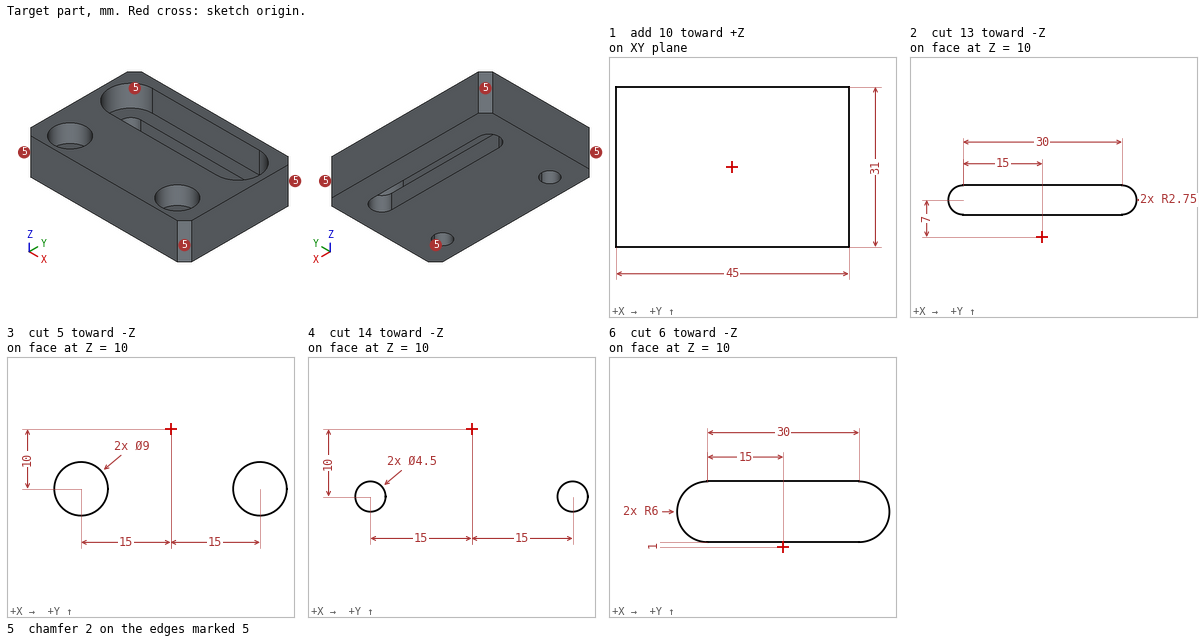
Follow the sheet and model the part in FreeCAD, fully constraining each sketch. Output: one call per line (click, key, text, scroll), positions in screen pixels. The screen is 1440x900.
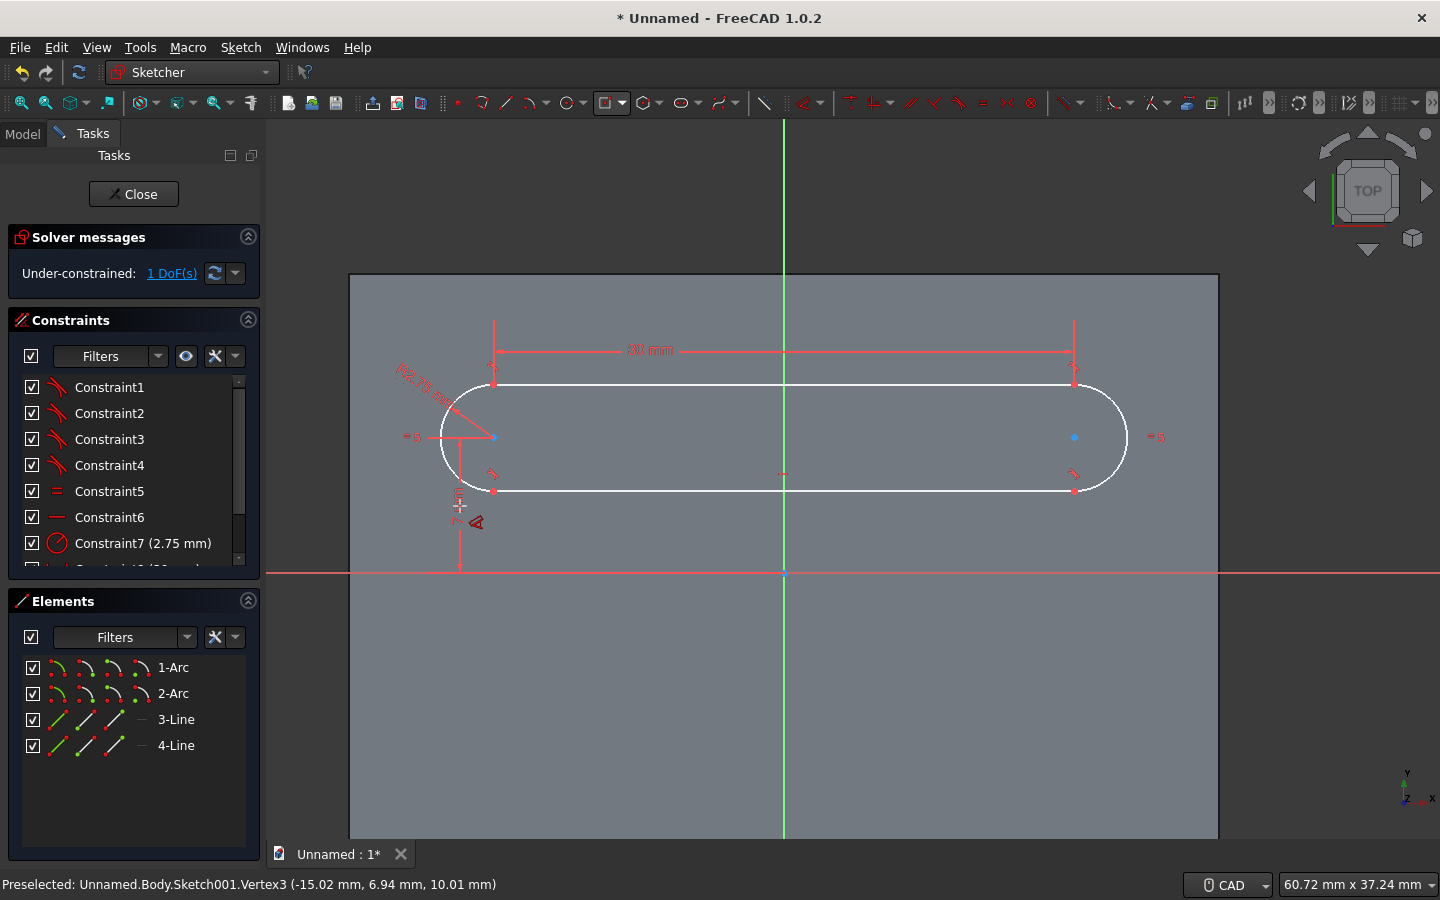
click(494, 385)
click(639, 607)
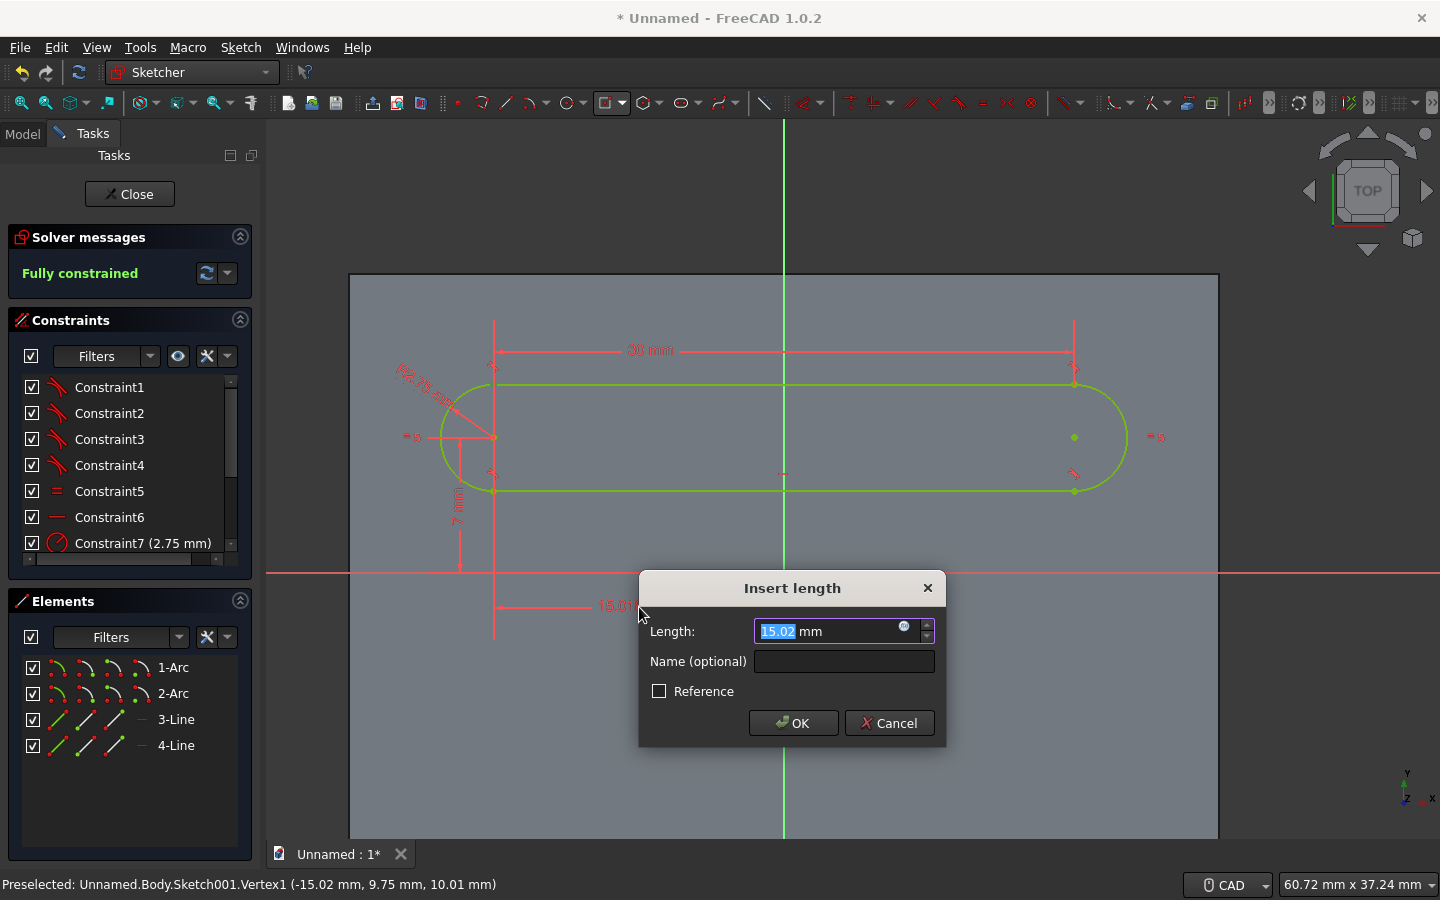
text(15)
key(Return)
key(Escape)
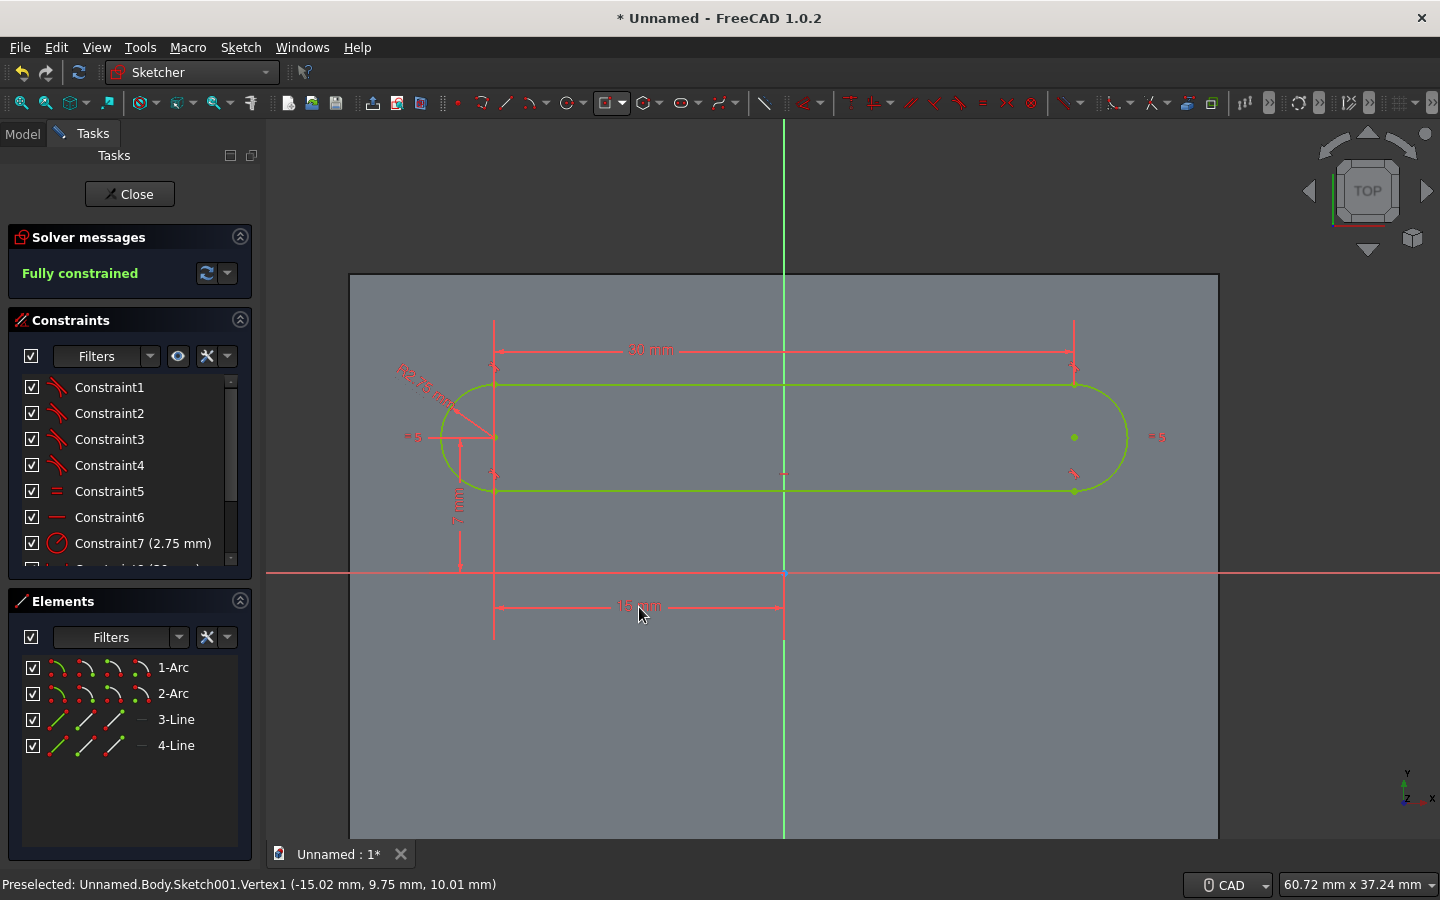
click(130, 194)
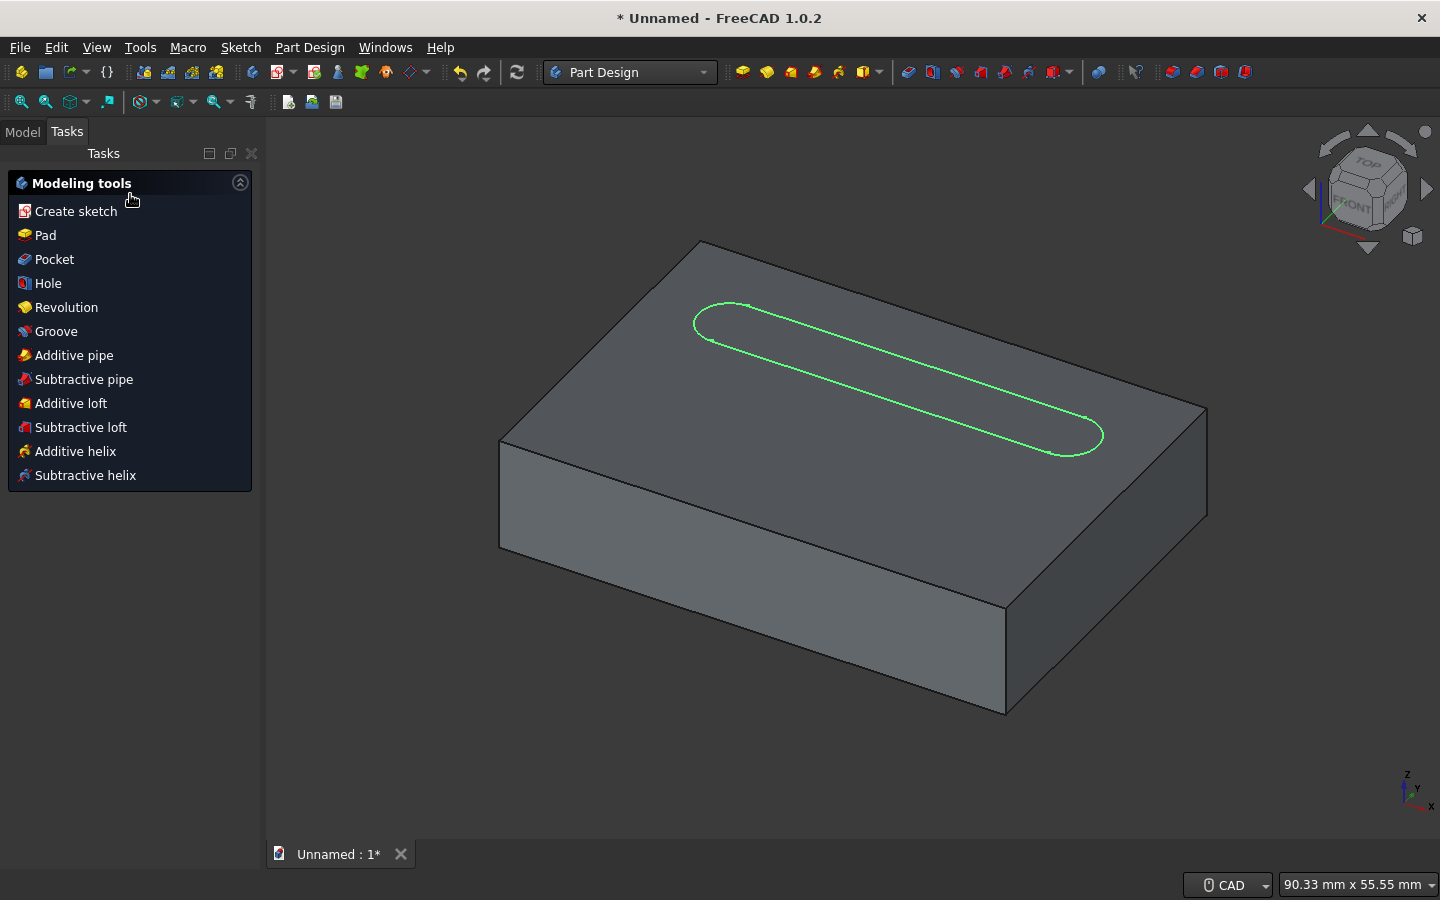
click(910, 72)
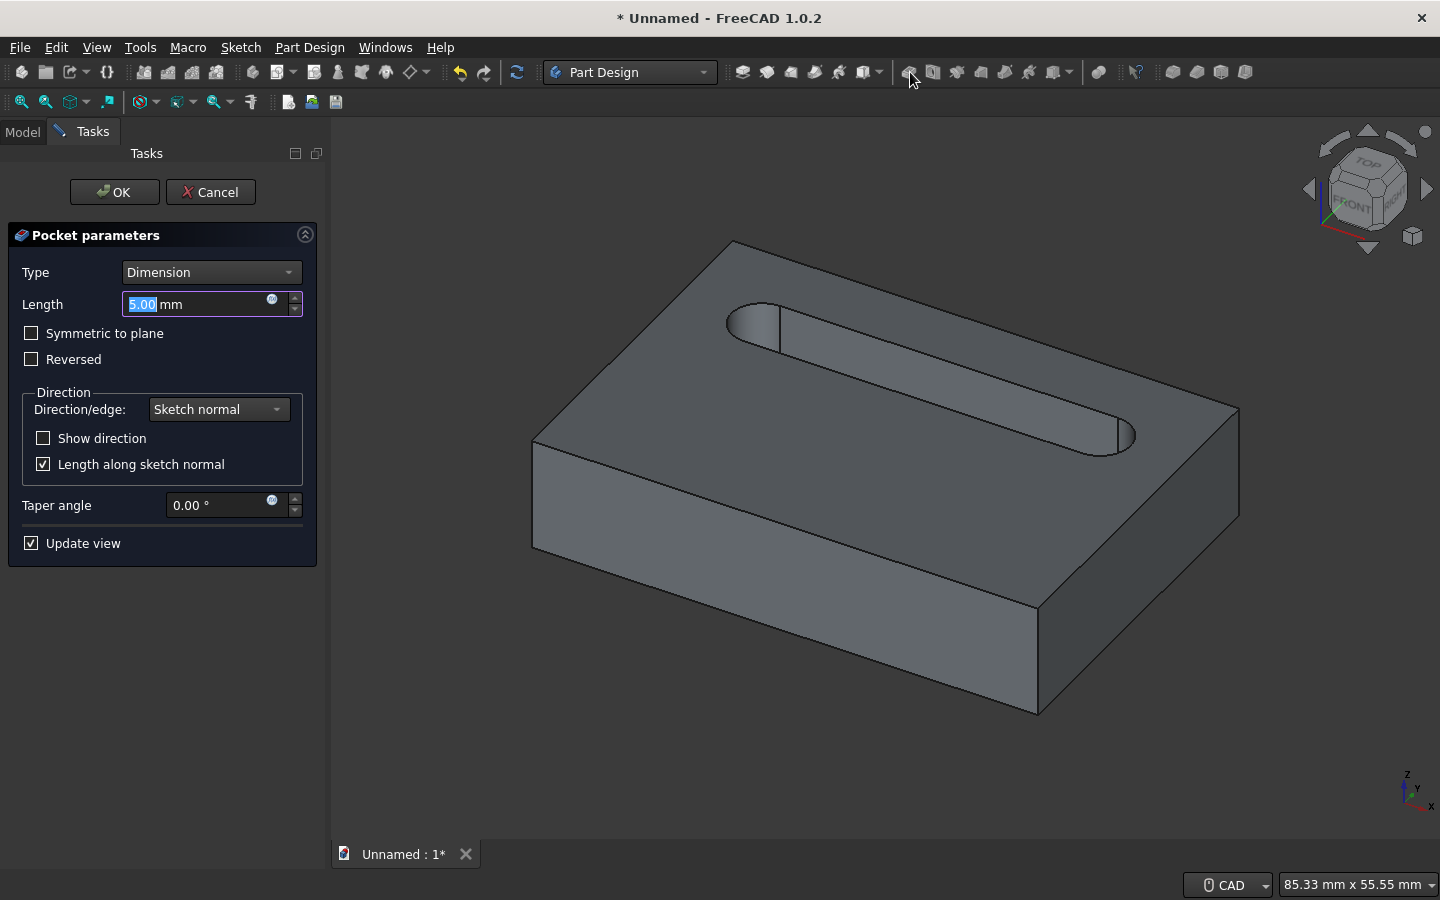
text(13)
key(Tab)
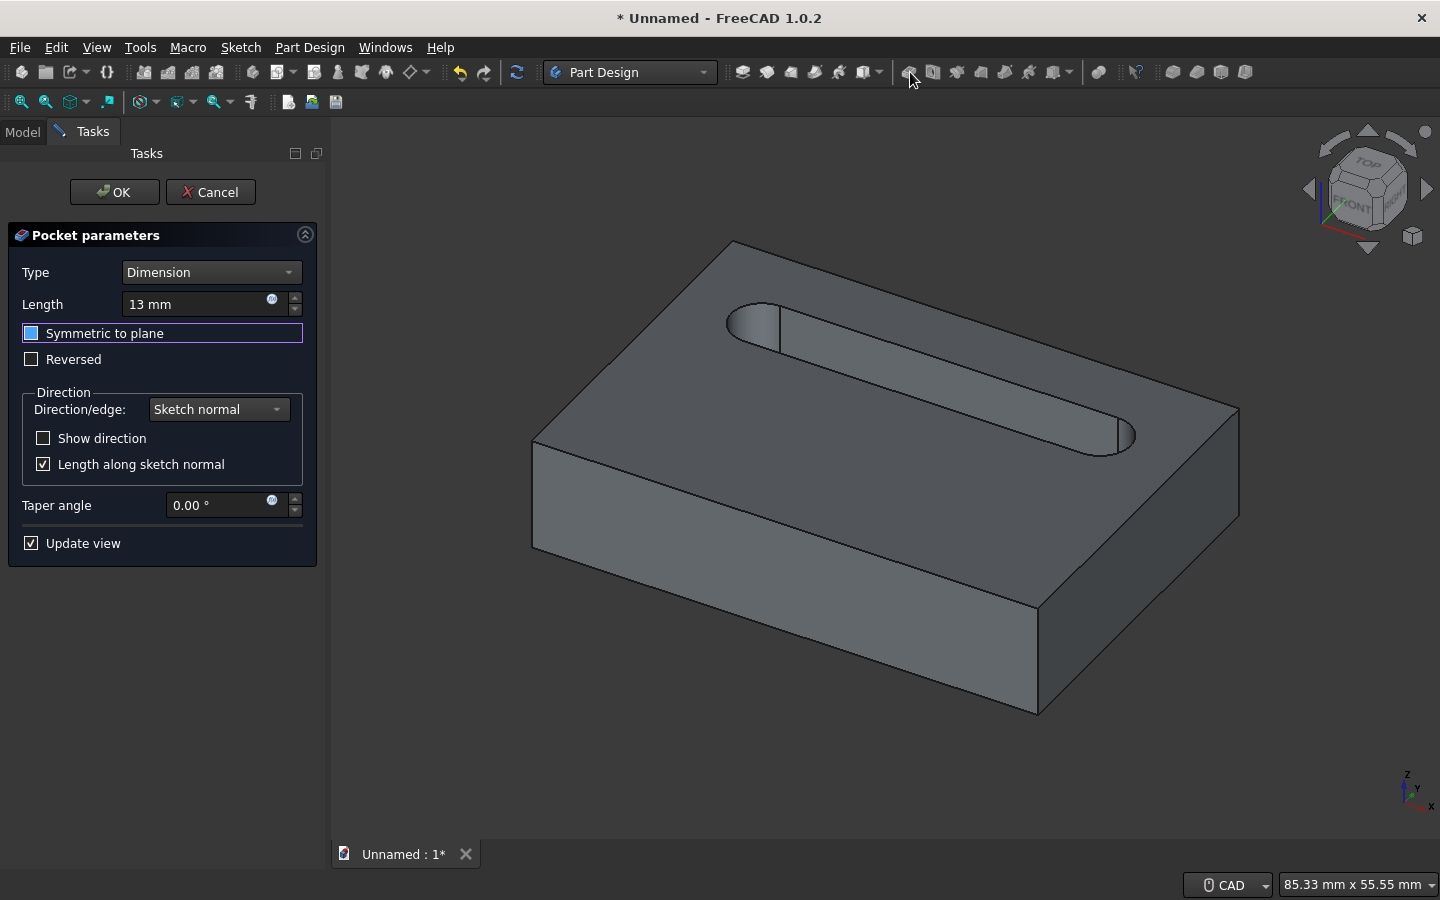
click(115, 192)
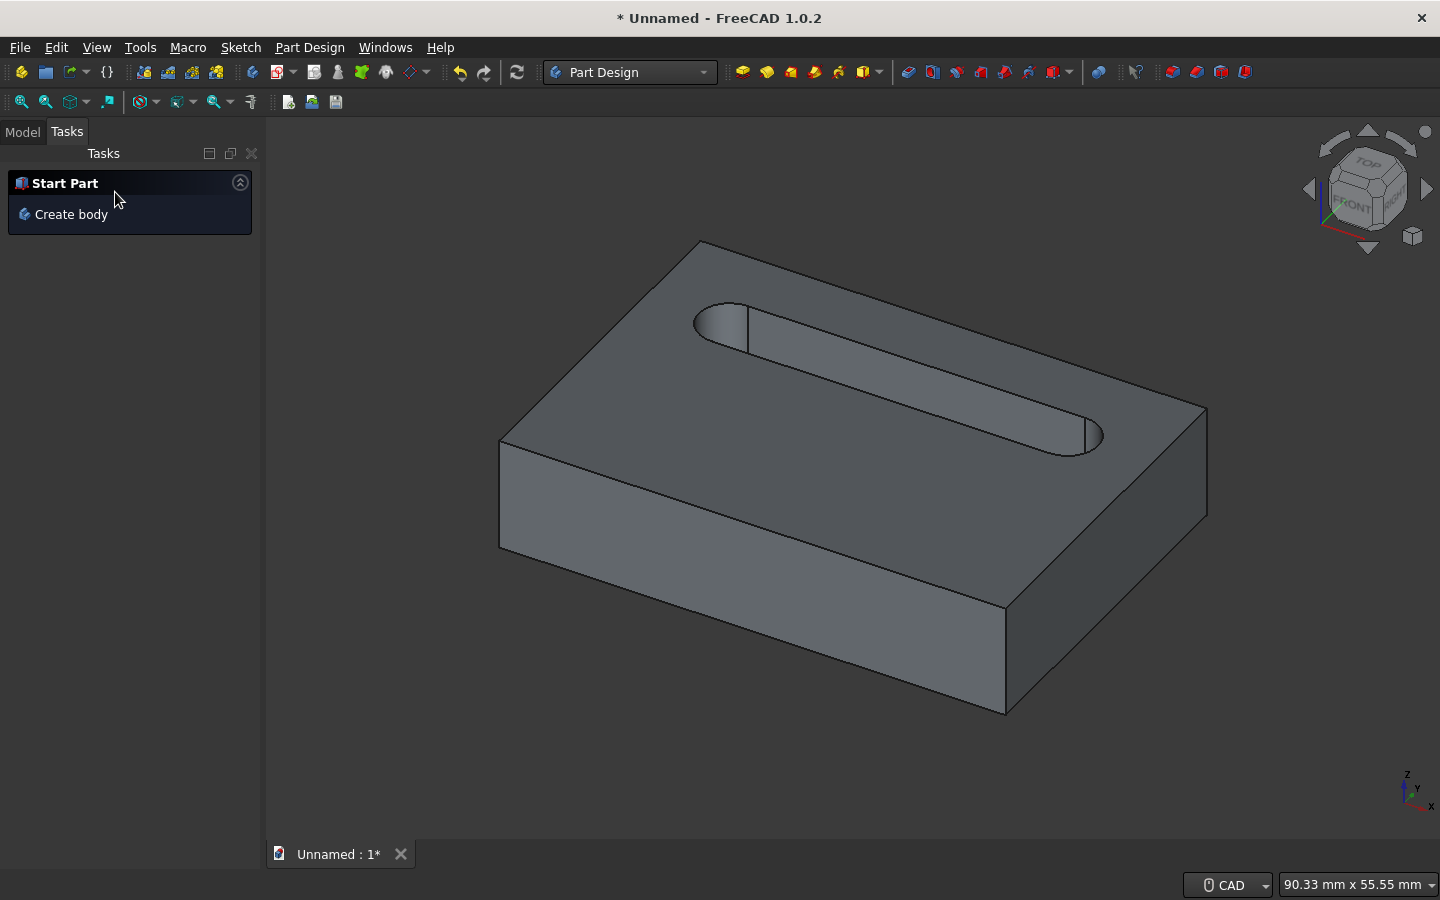
click(969, 500)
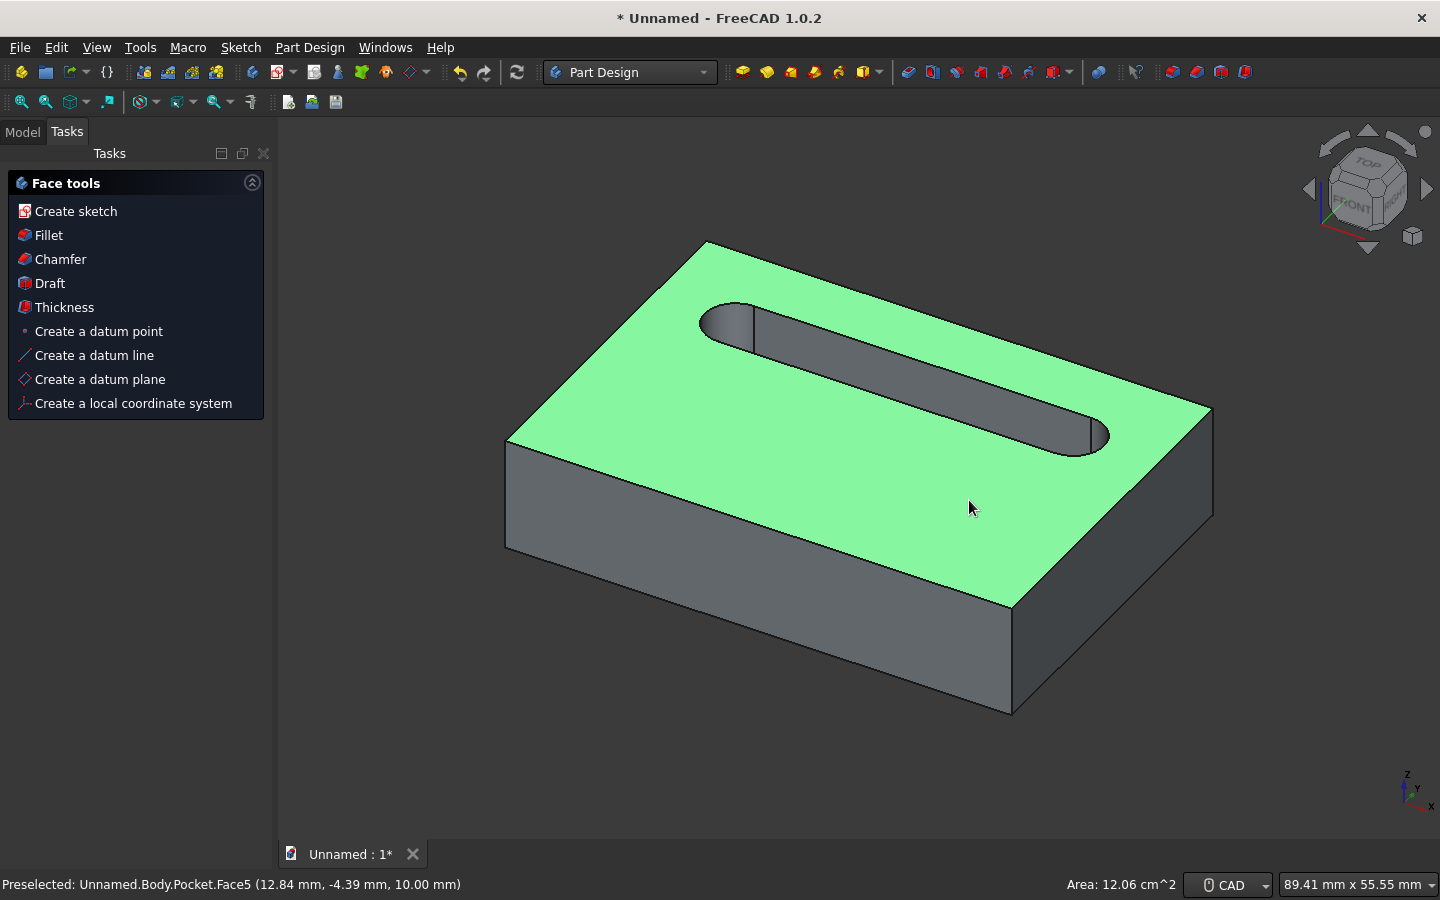
click(278, 72)